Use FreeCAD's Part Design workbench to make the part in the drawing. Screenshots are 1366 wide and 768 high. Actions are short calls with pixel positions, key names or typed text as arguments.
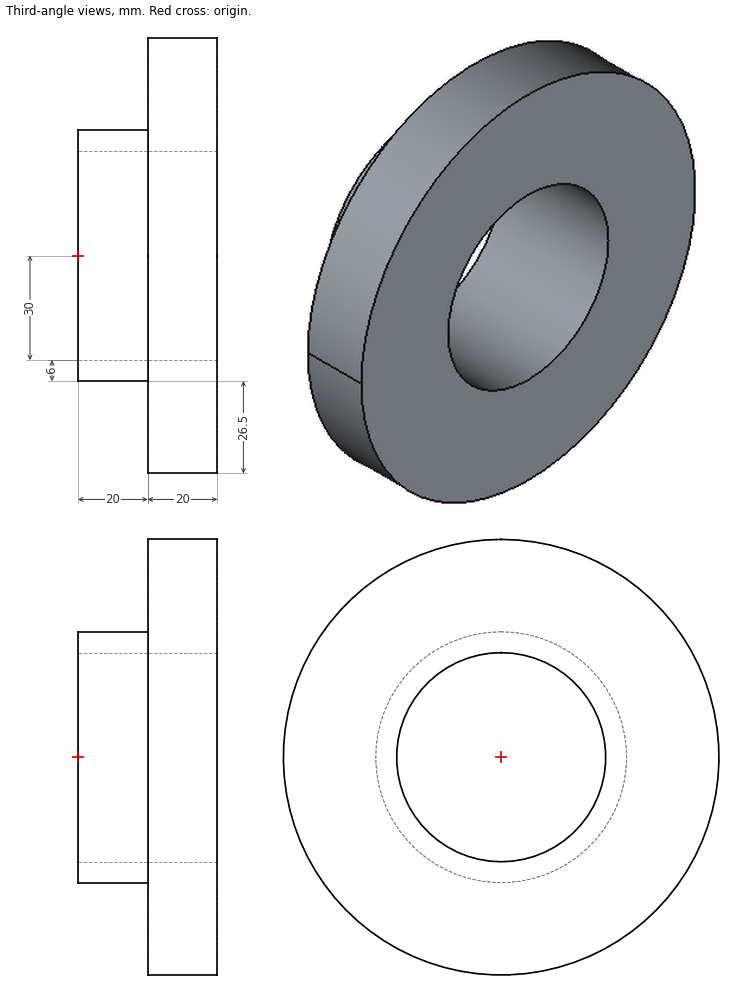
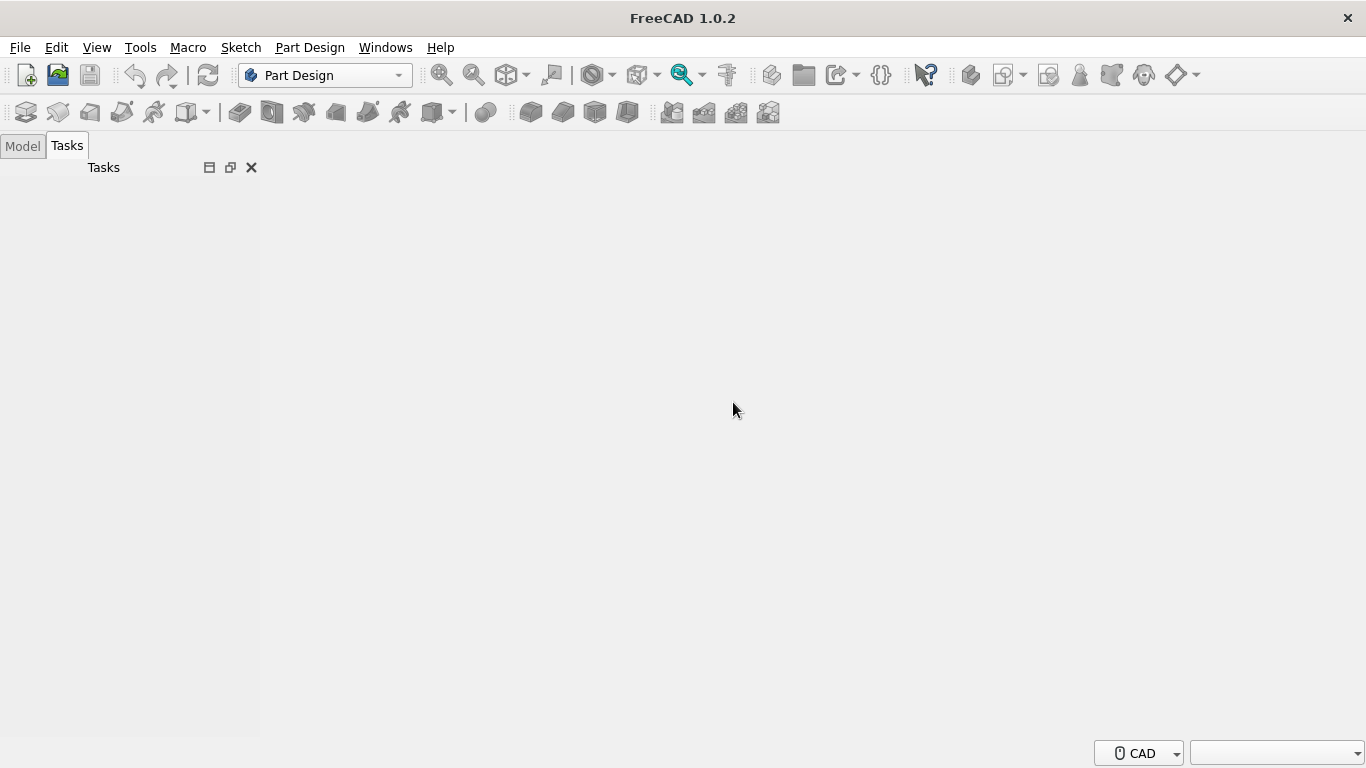
click(26, 76)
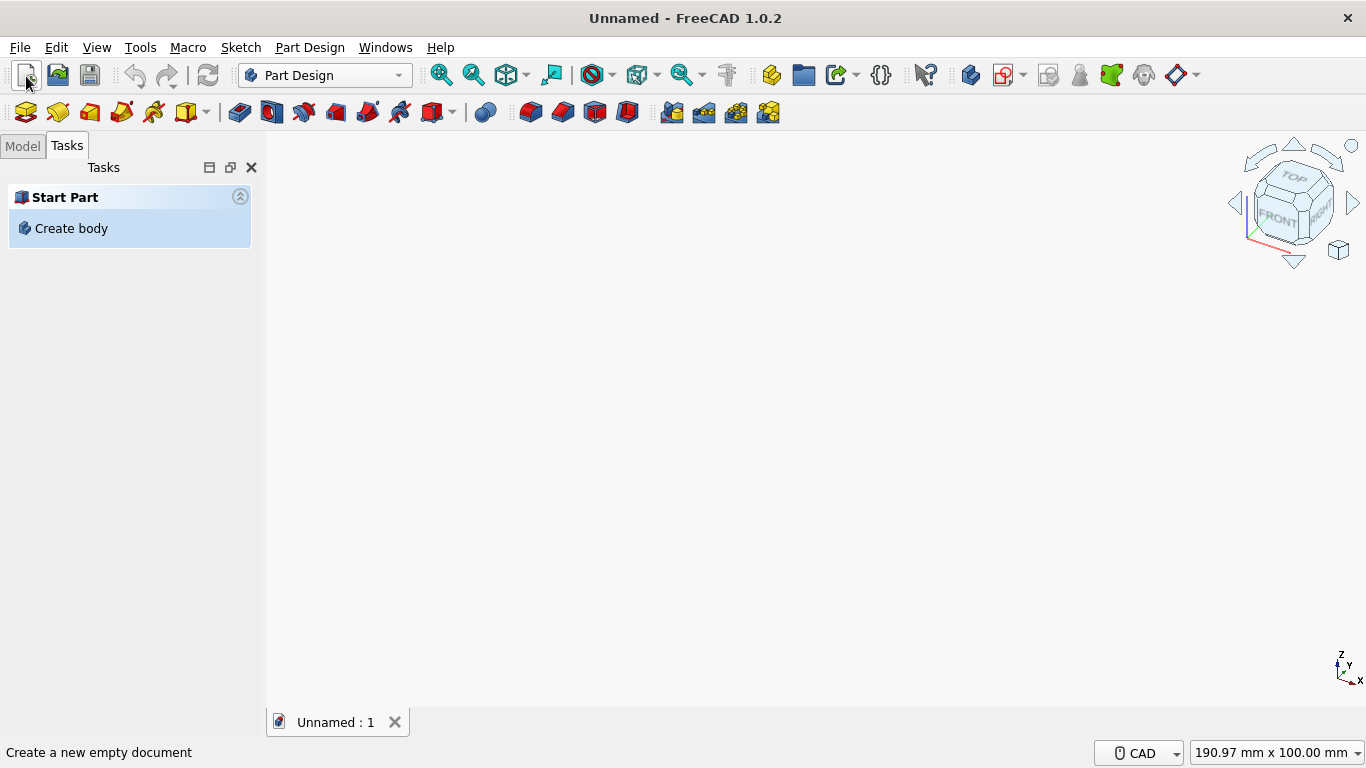
click(1004, 76)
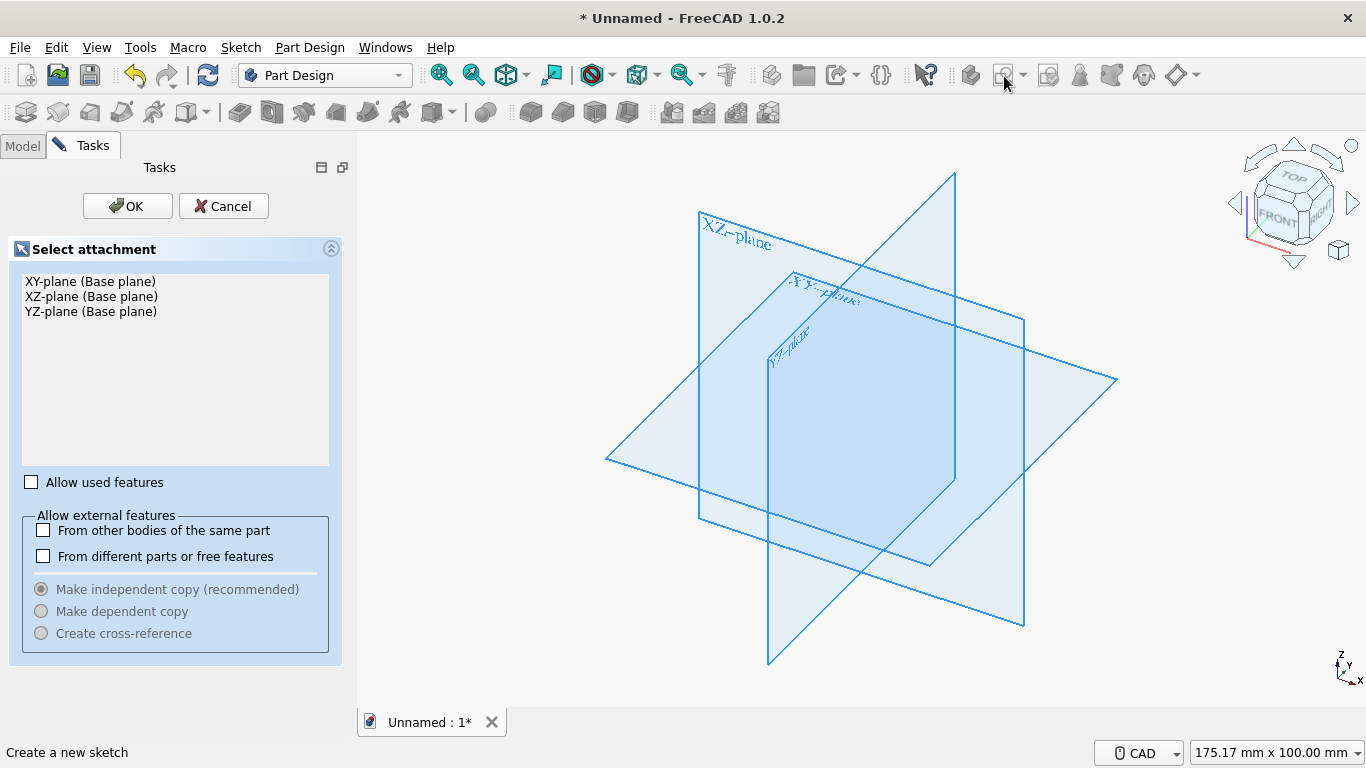
click(82, 282)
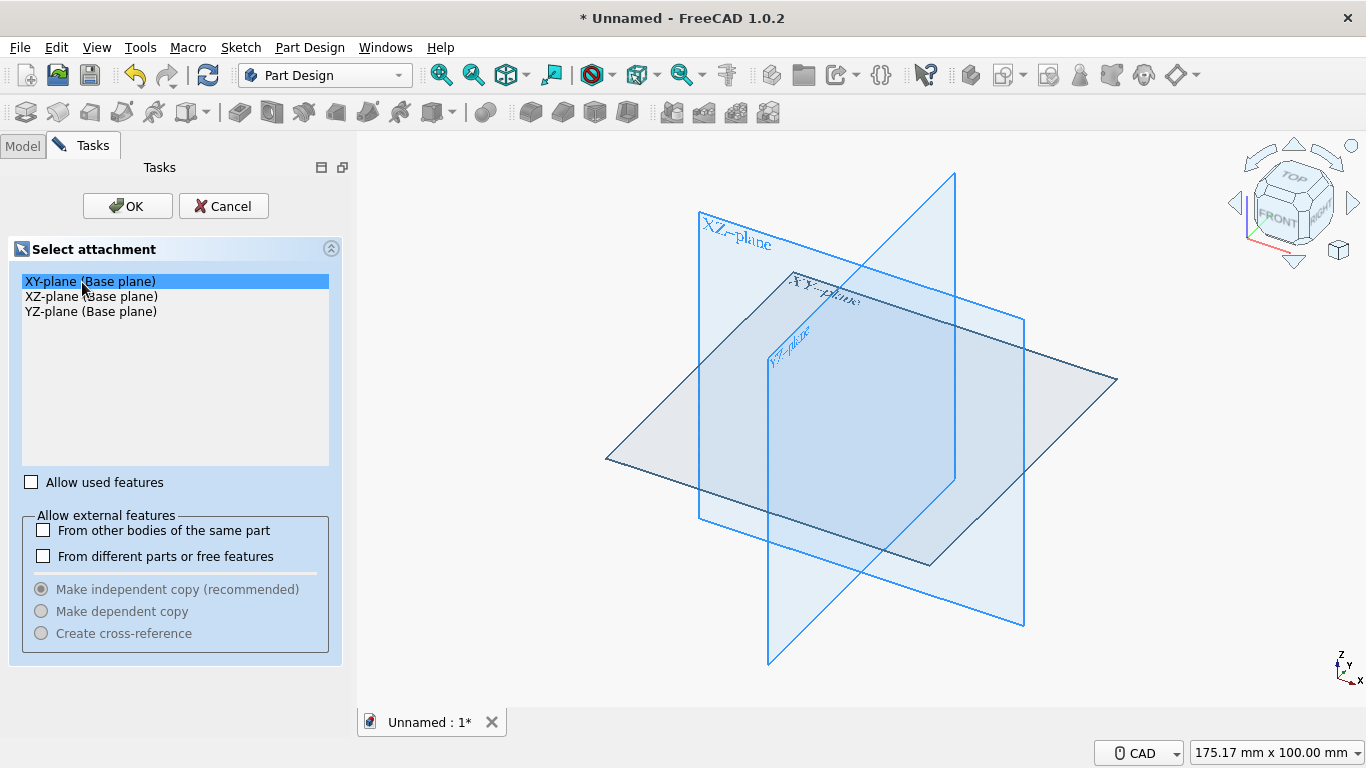
click(128, 206)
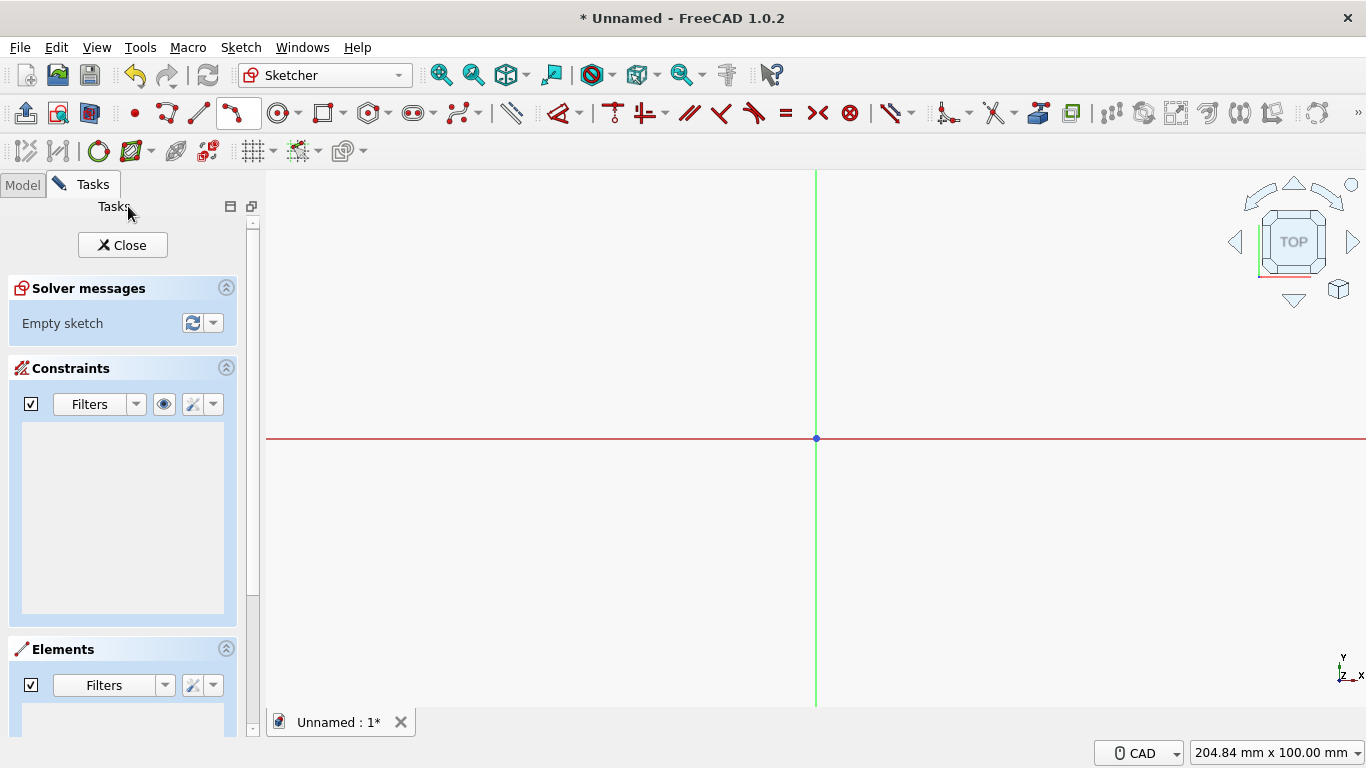
scroll(390, 198, down, 2)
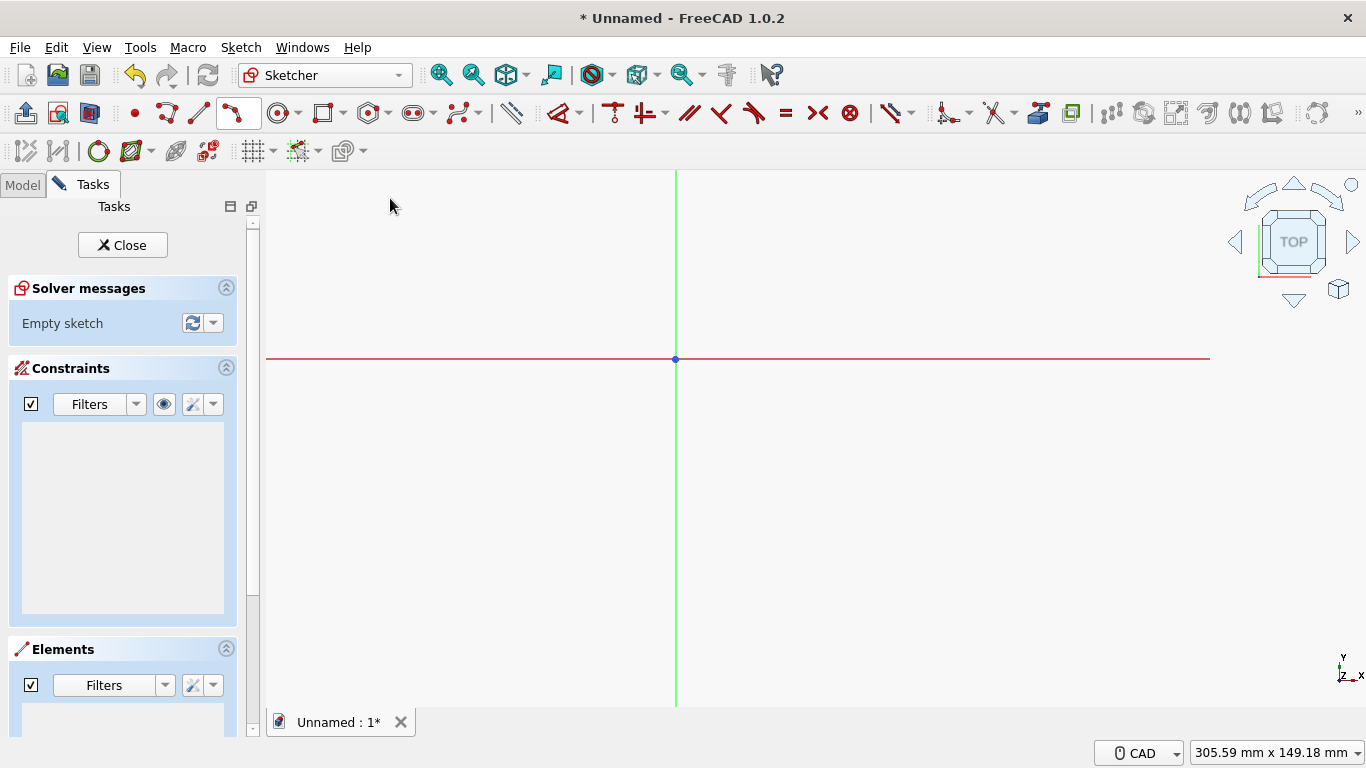
scroll(748, 539, up, 2)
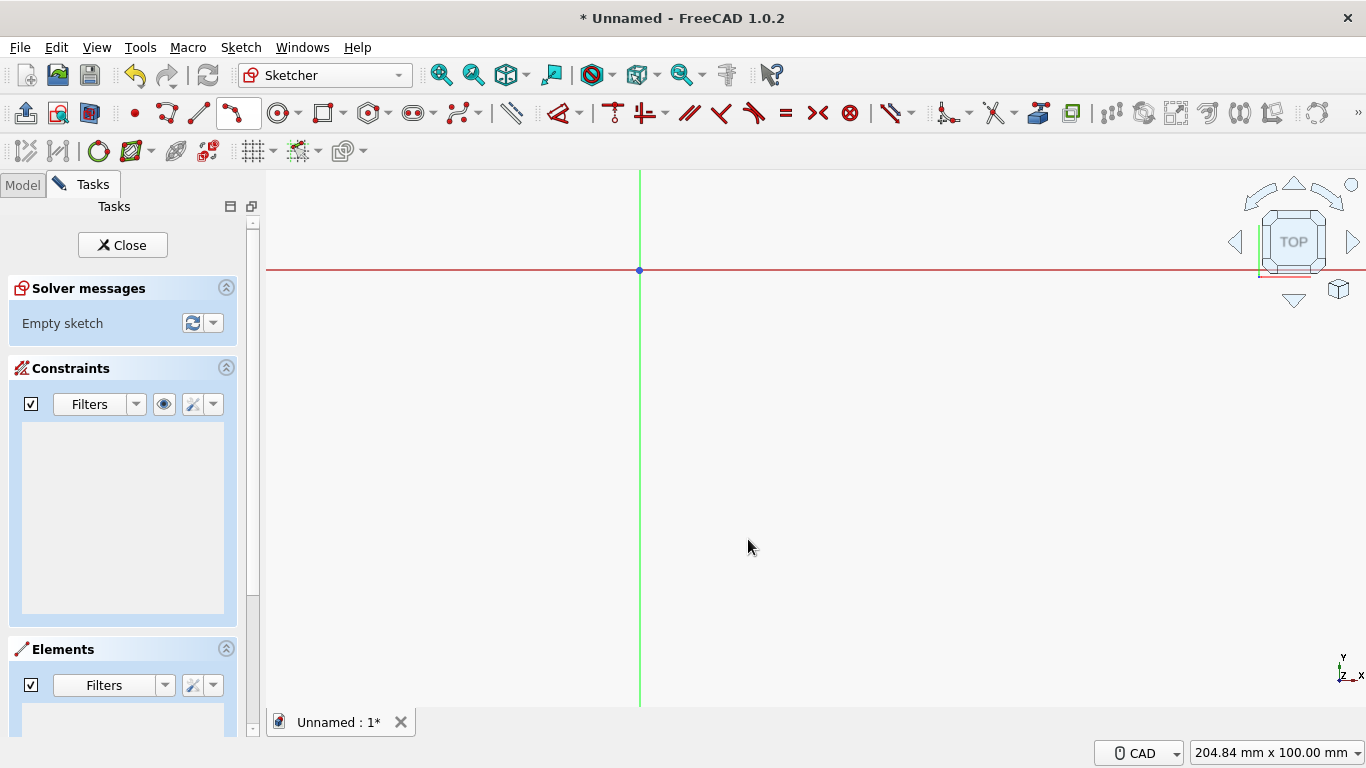
click(168, 114)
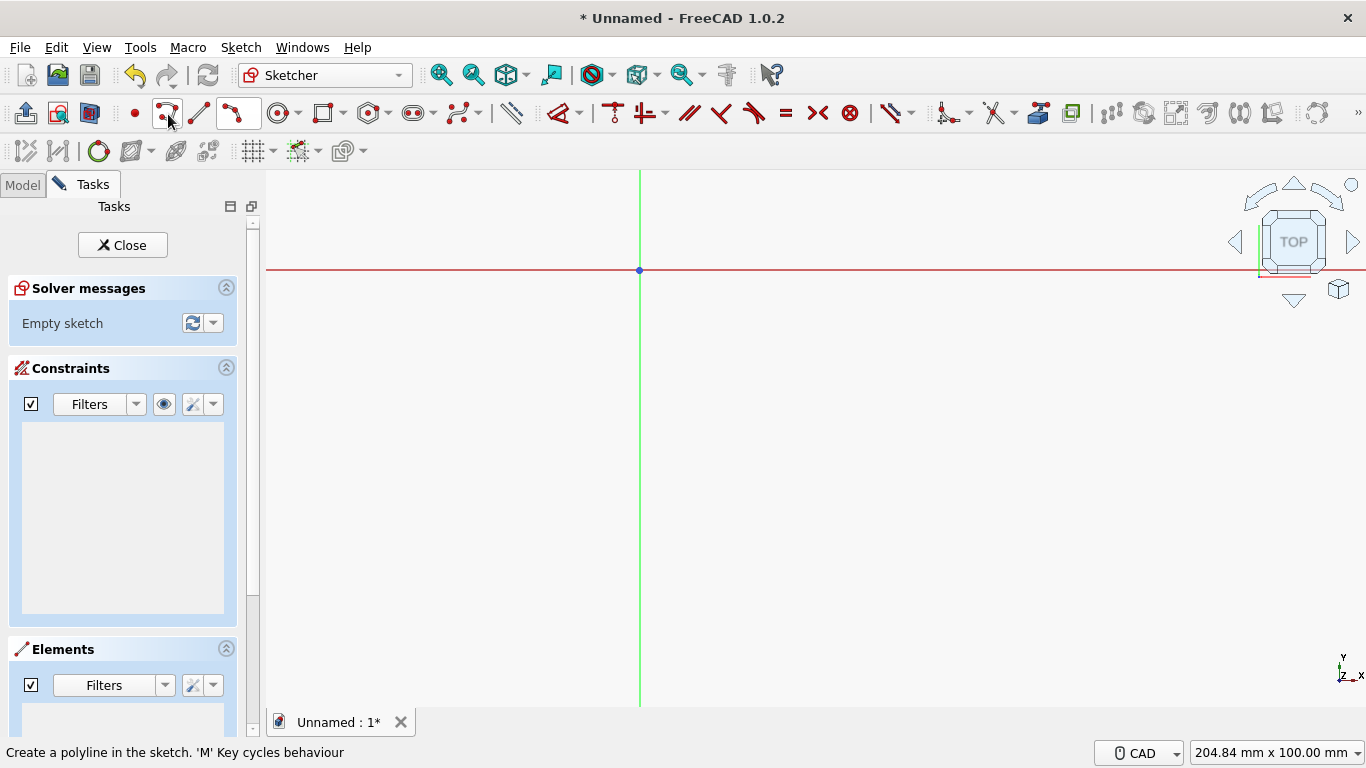
click(640, 432)
click(649, 464)
click(747, 464)
click(747, 606)
click(855, 606)
click(855, 432)
click(640, 433)
key(Escape)
key(Escape)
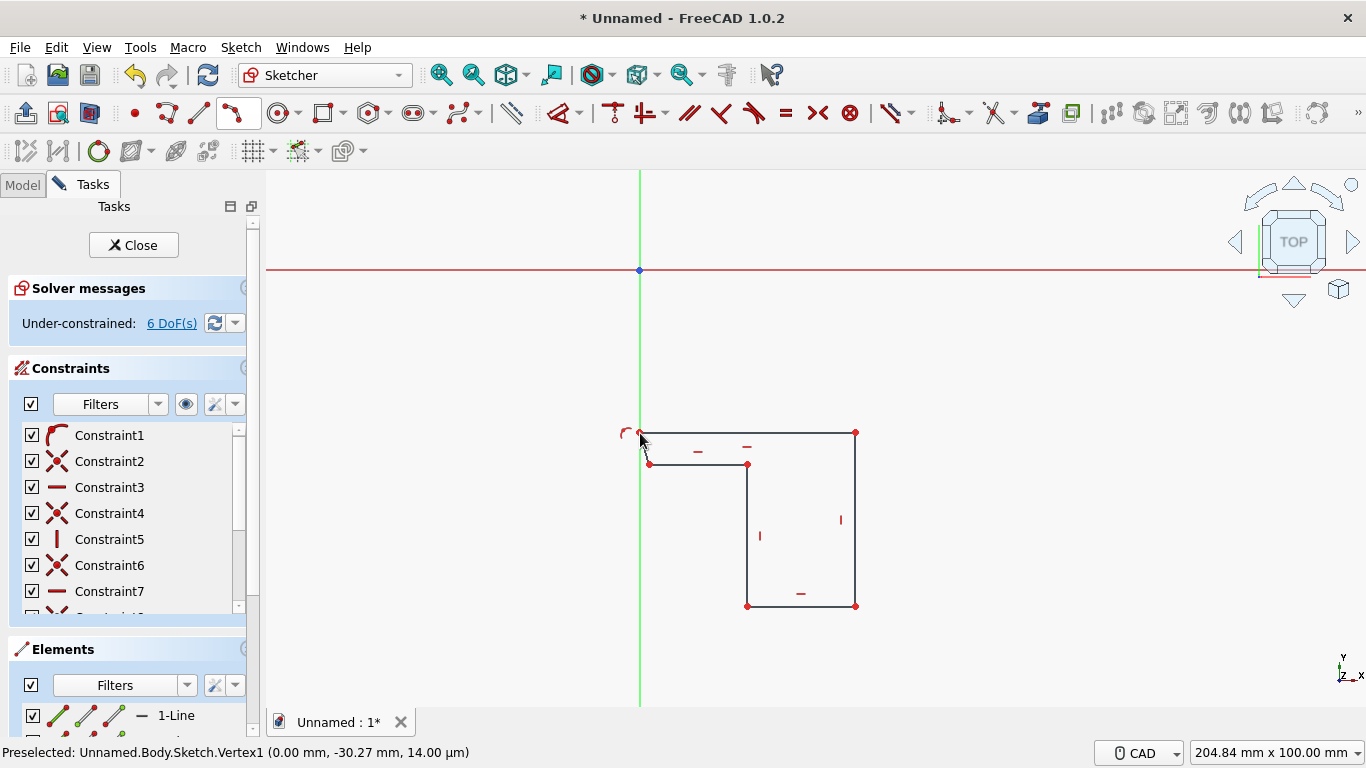
scroll(643, 443, up, 2)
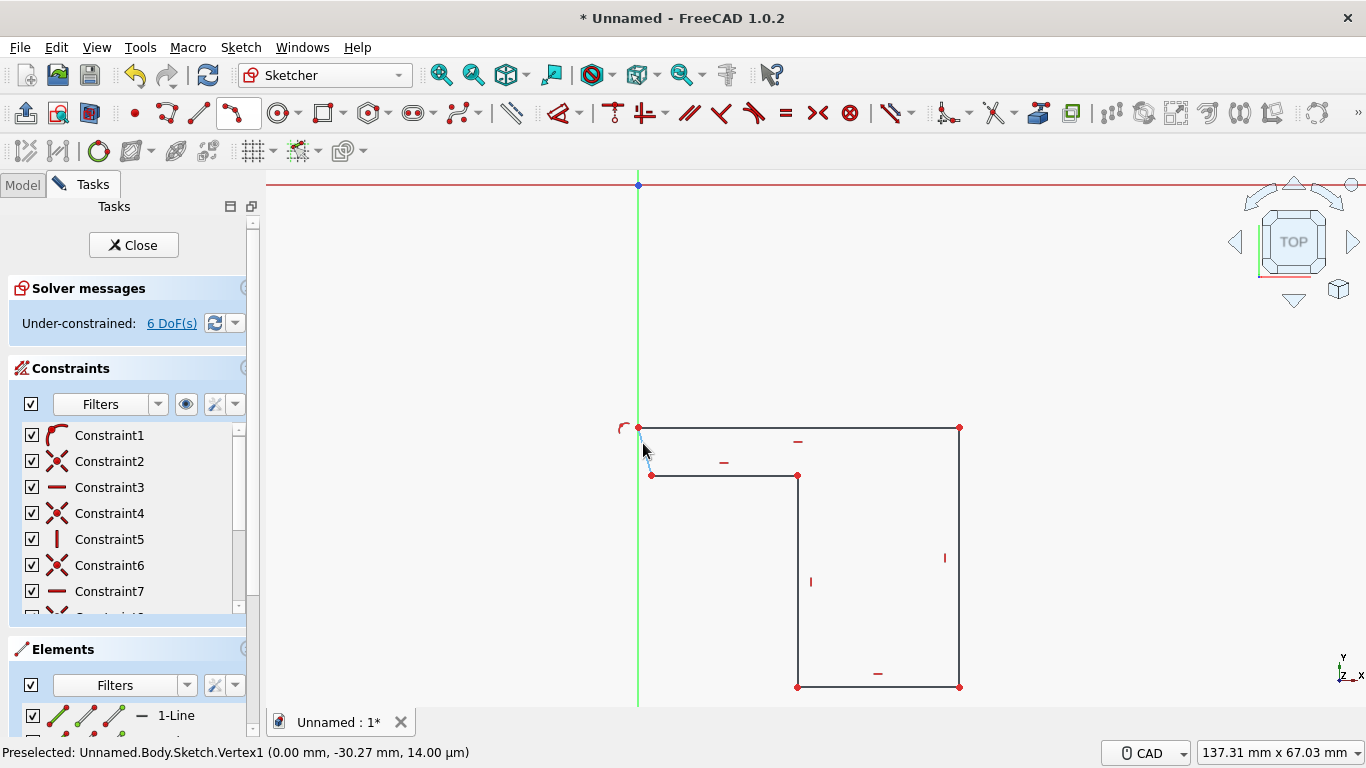
click(642, 442)